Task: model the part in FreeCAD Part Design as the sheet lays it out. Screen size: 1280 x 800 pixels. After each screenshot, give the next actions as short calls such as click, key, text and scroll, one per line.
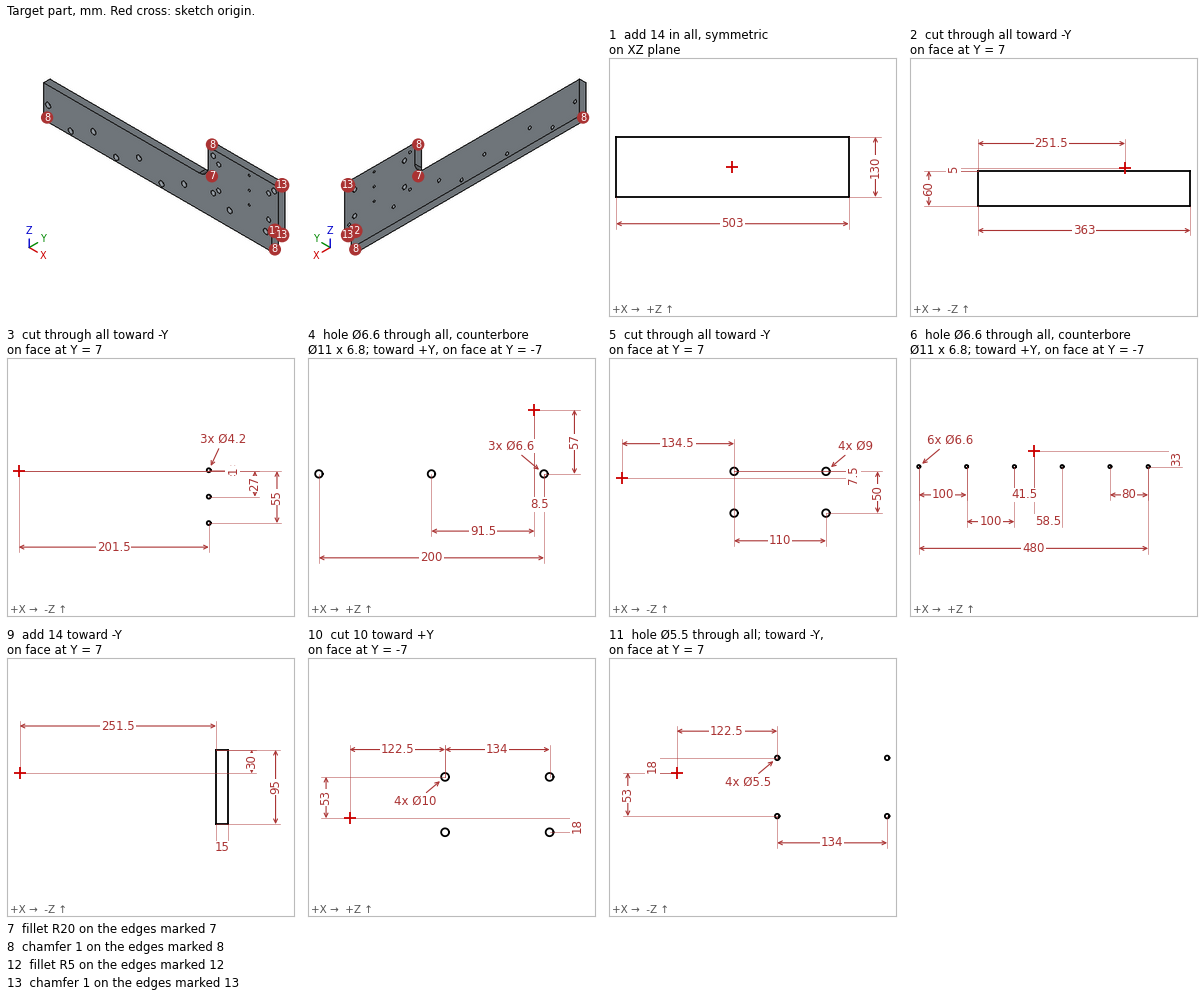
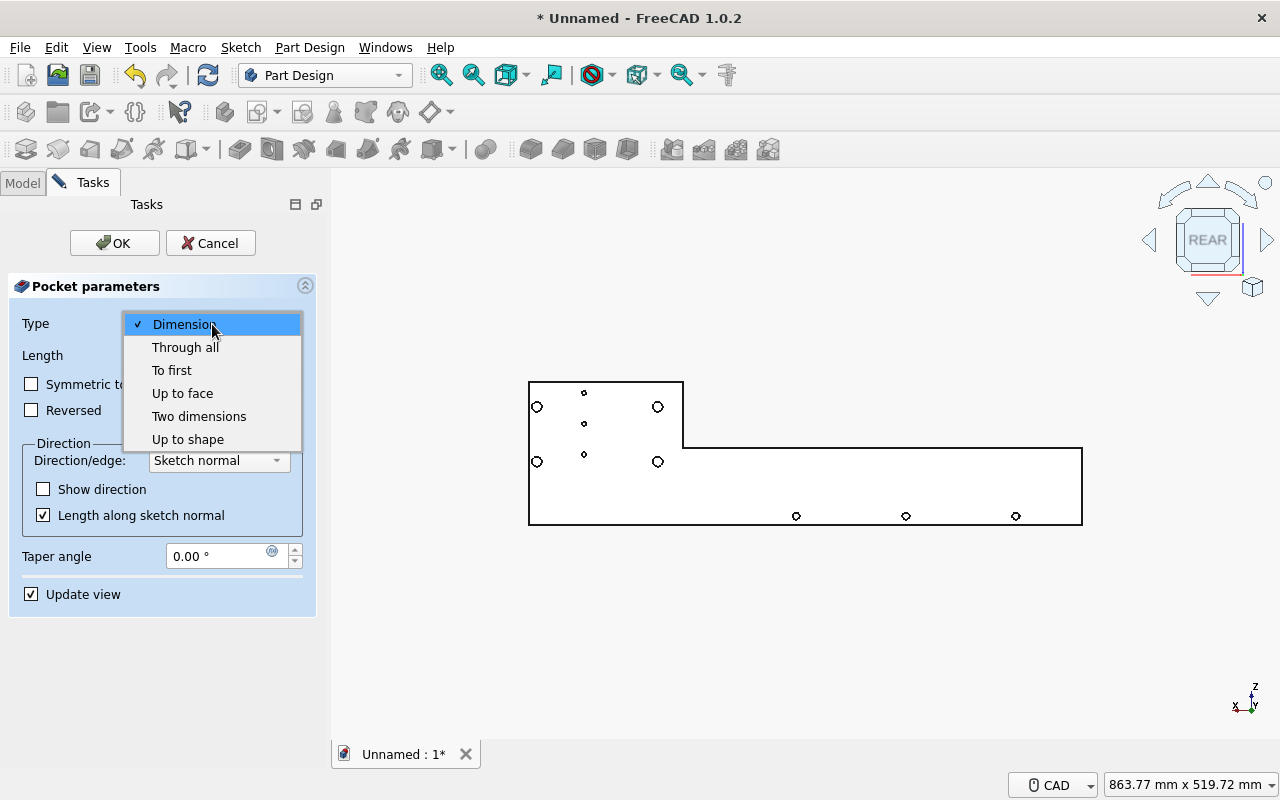
click(212, 348)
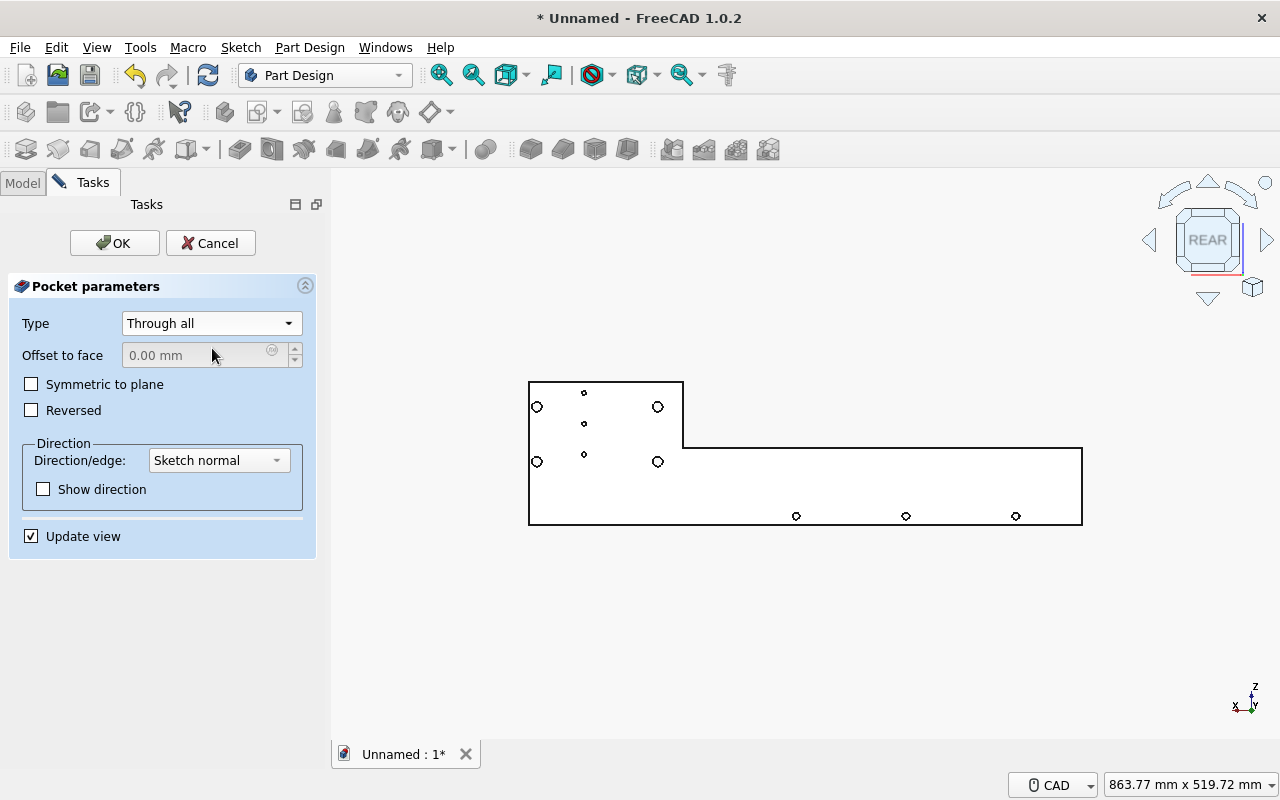
click(115, 243)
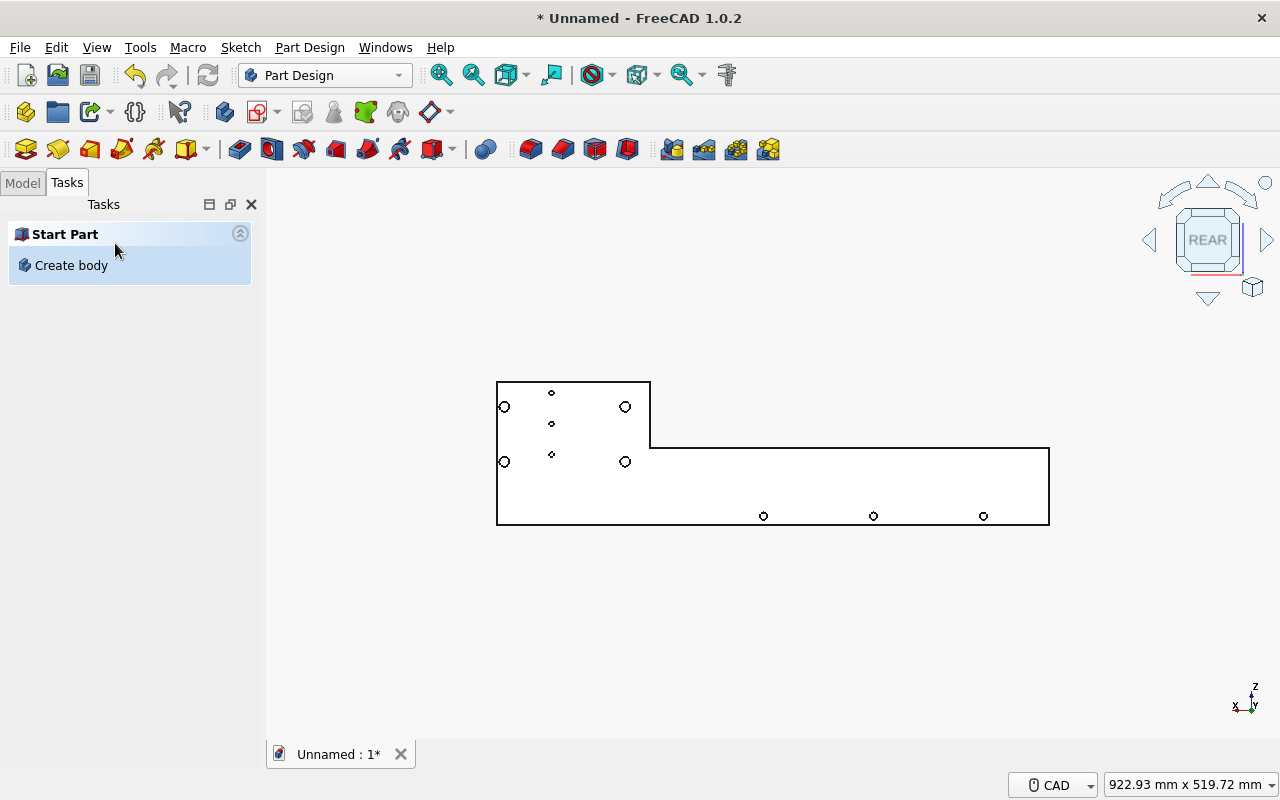
key(0)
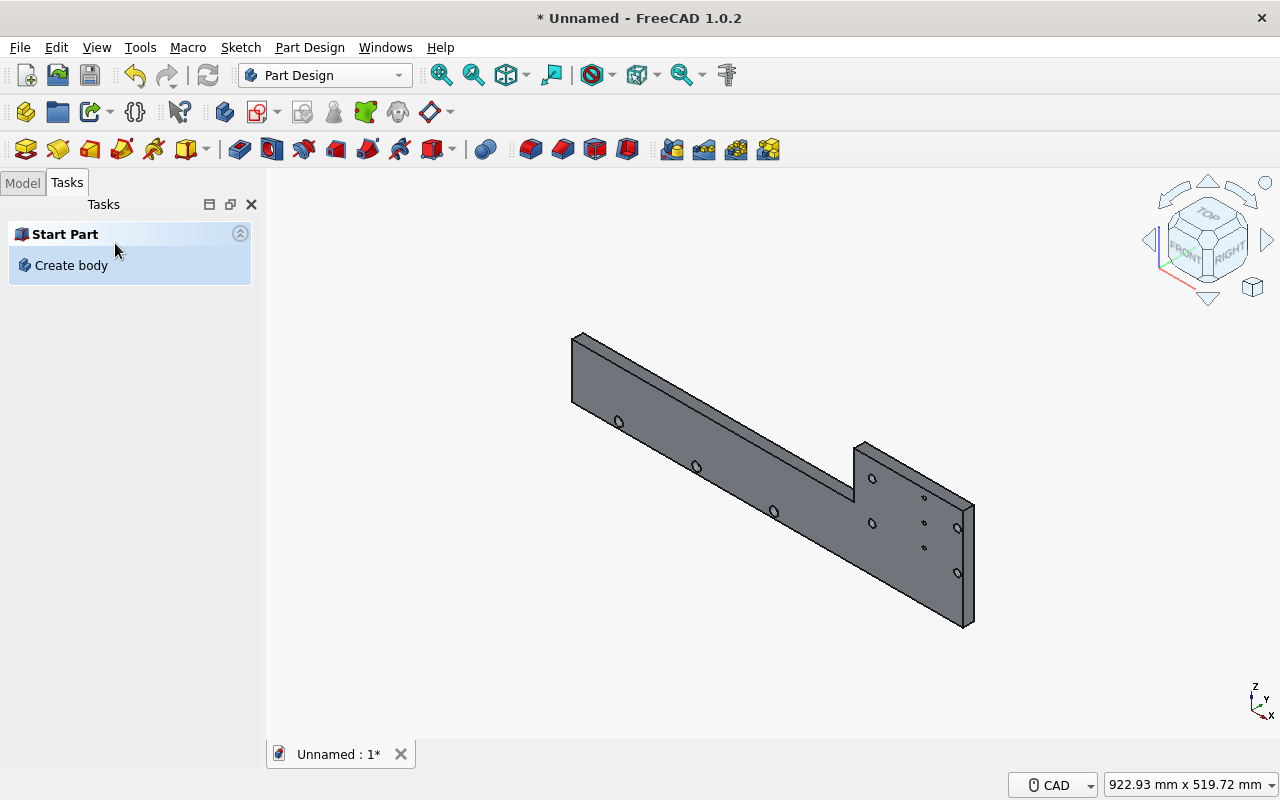
click(935, 586)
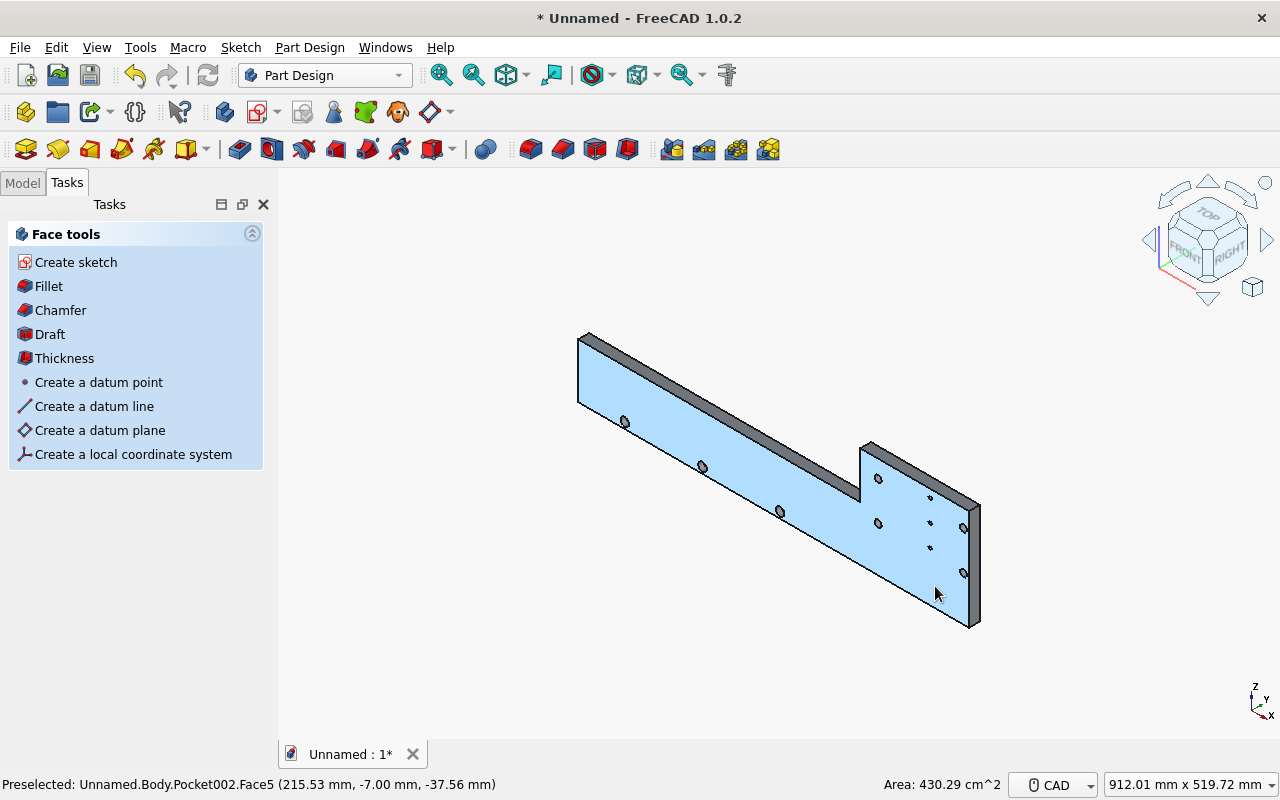
click(258, 112)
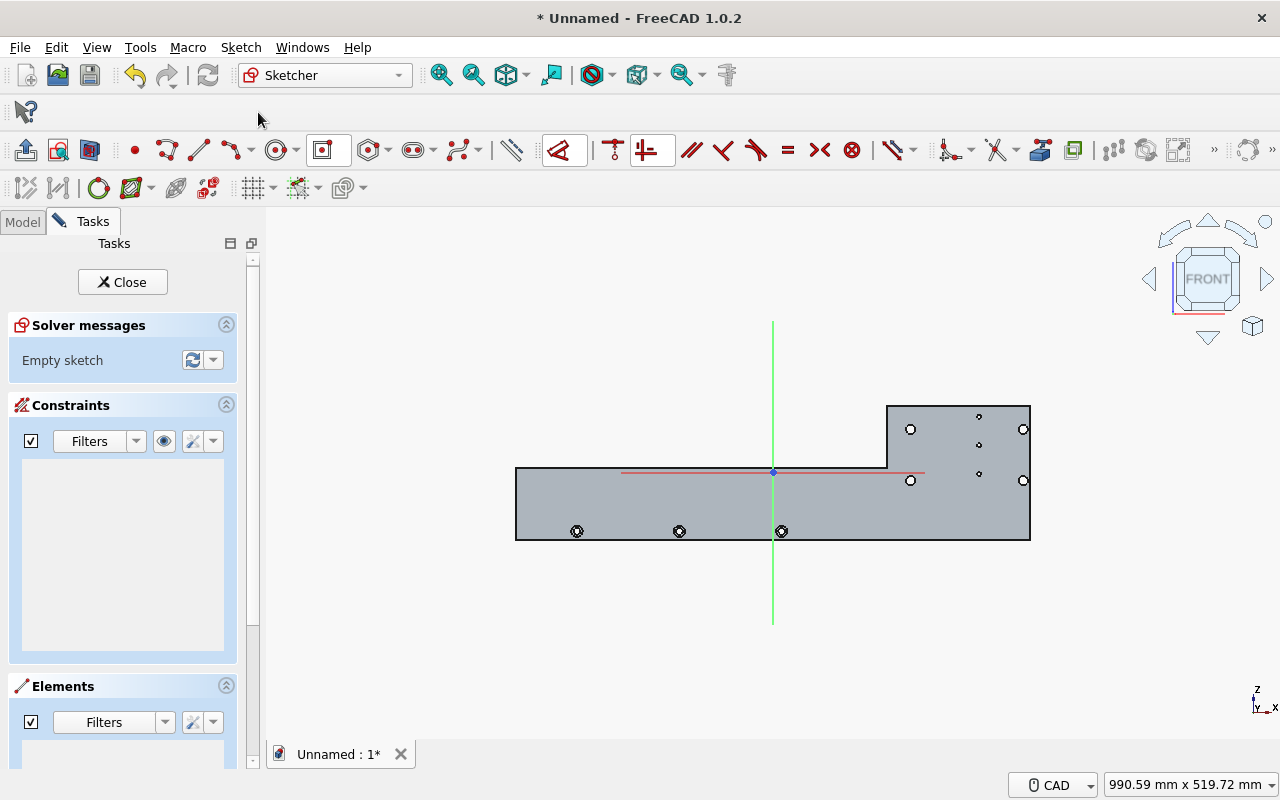
key(g)
key(c)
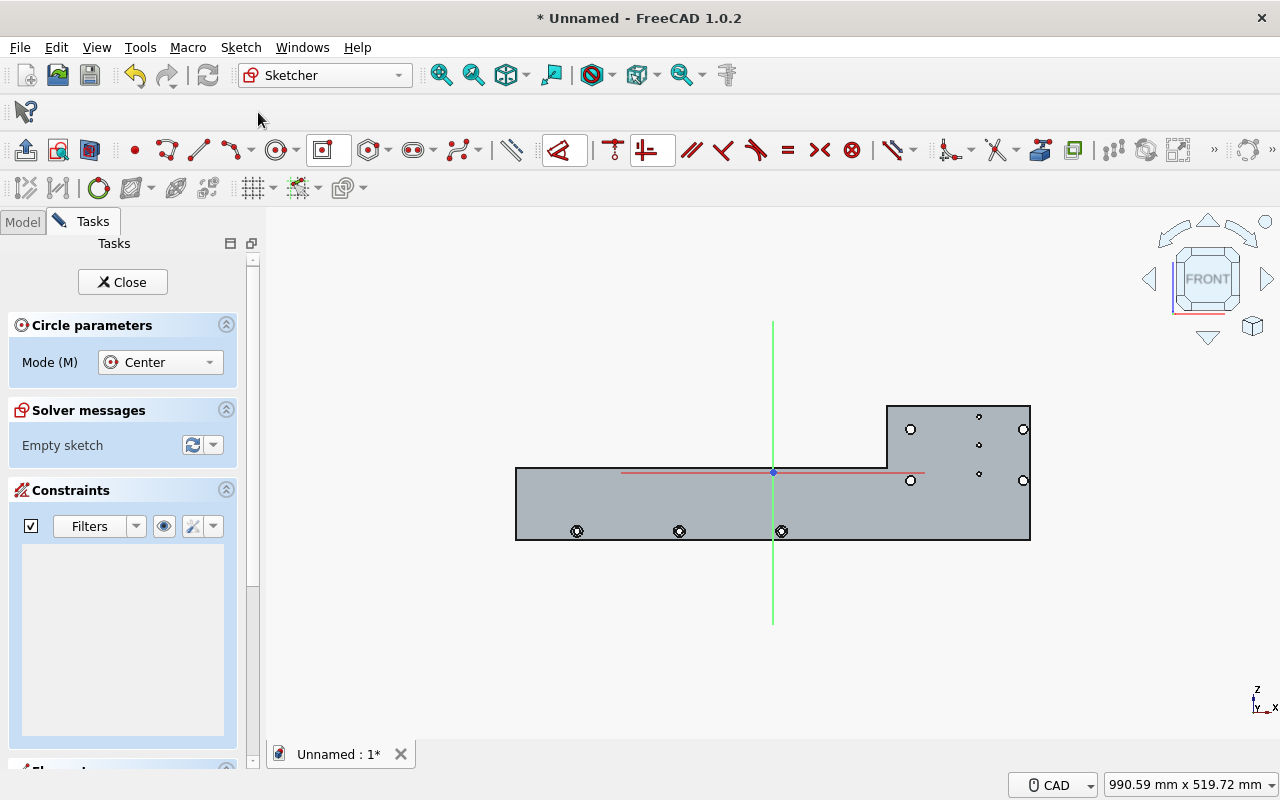
scroll(1017, 507, up, 10)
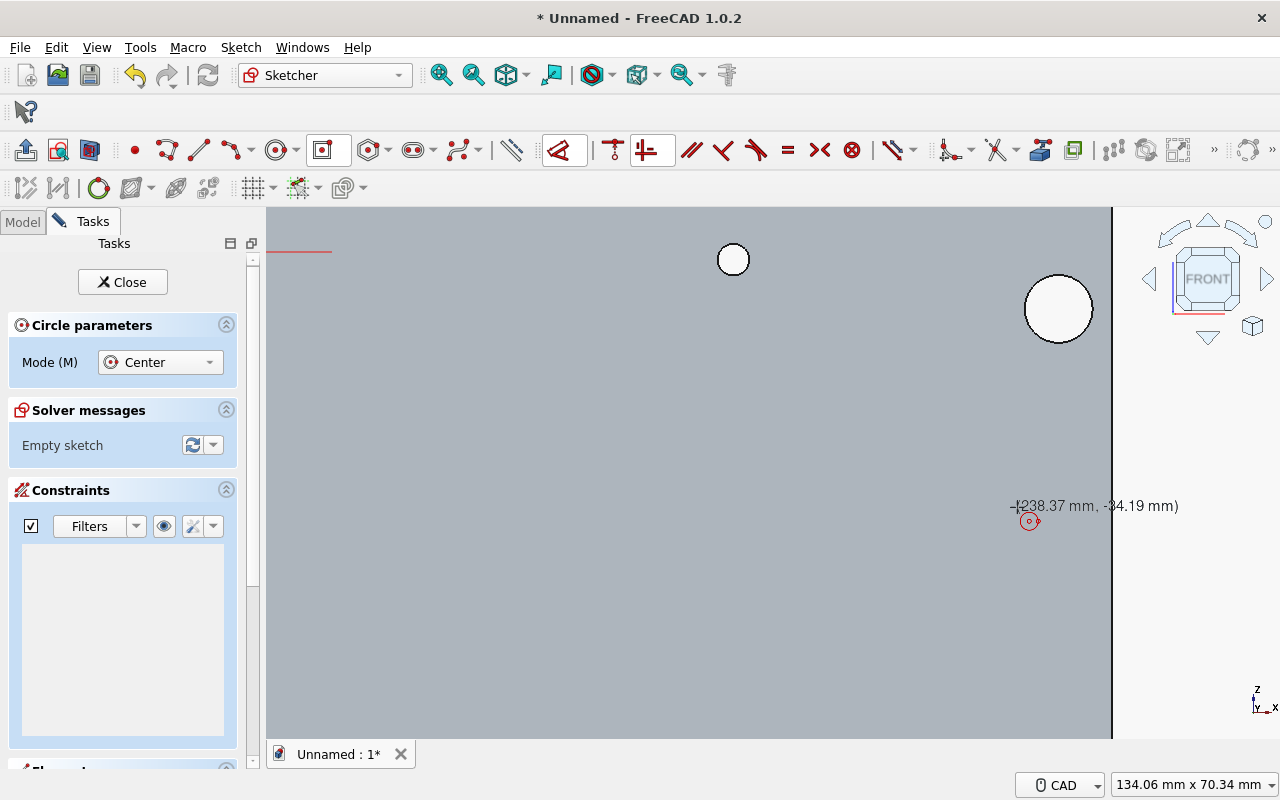
scroll(1003, 490, down, 9)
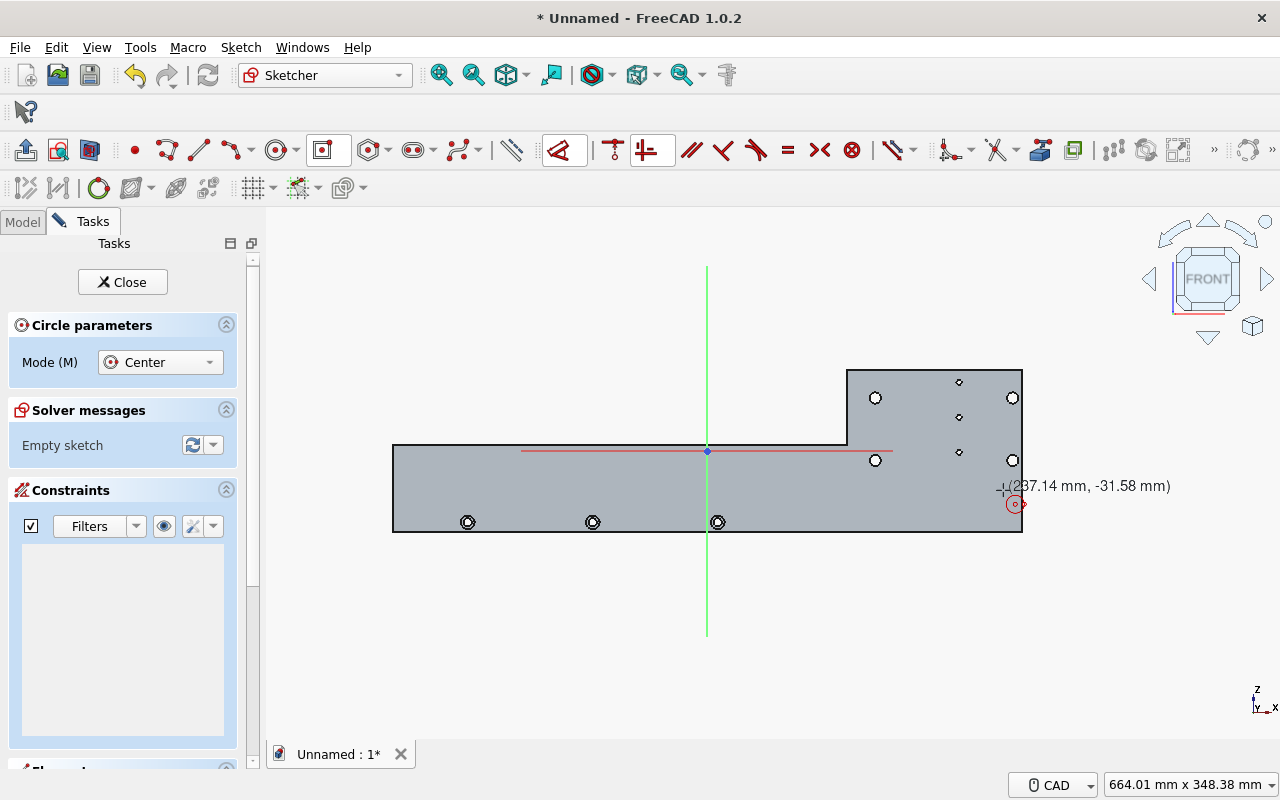
click(1005, 492)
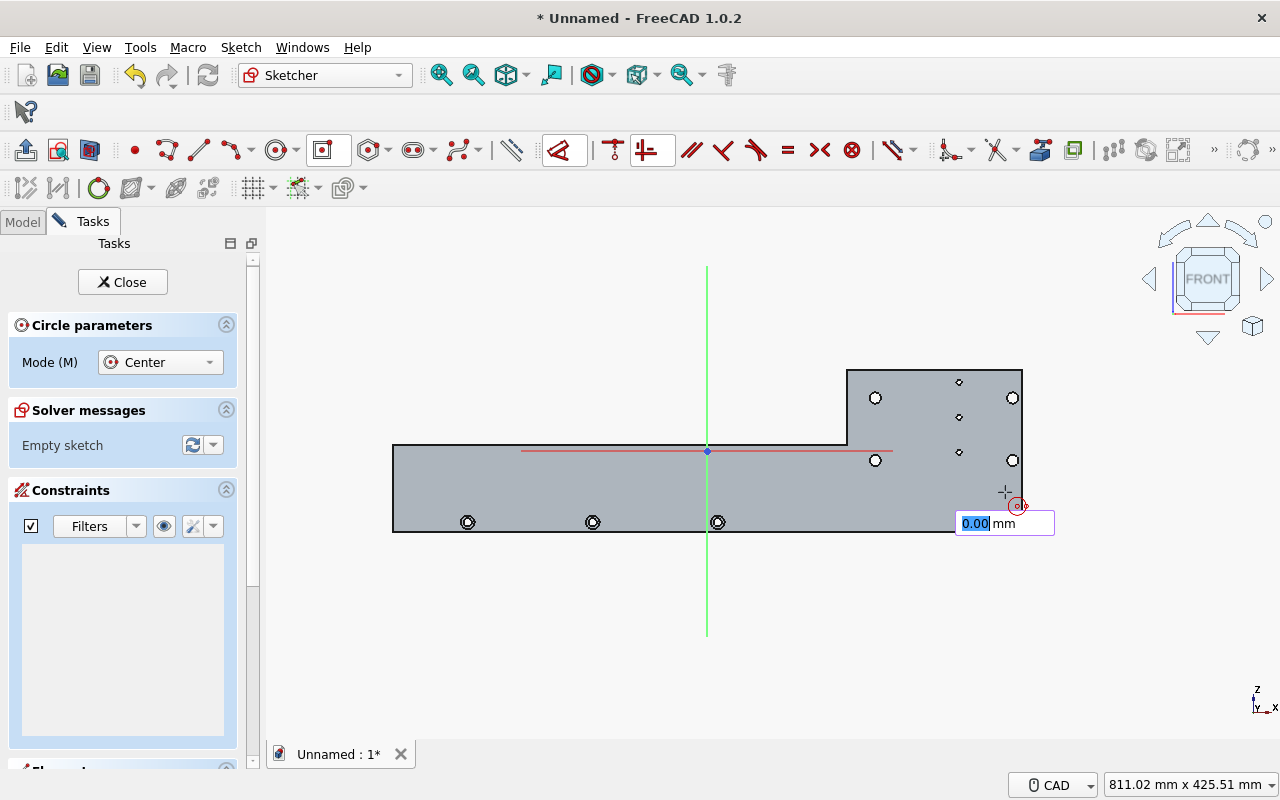
scroll(1008, 489, up, 7)